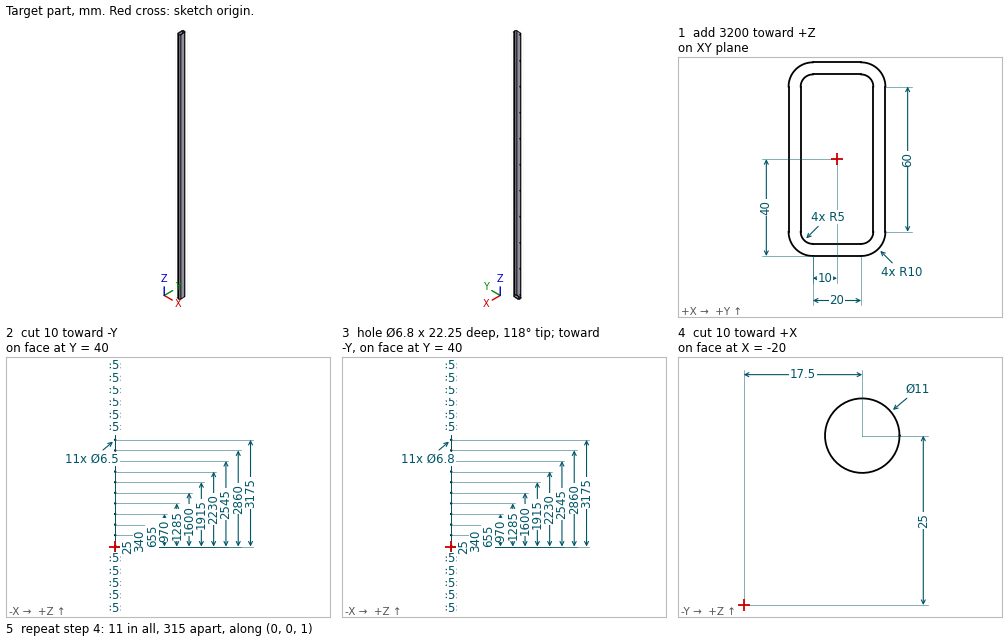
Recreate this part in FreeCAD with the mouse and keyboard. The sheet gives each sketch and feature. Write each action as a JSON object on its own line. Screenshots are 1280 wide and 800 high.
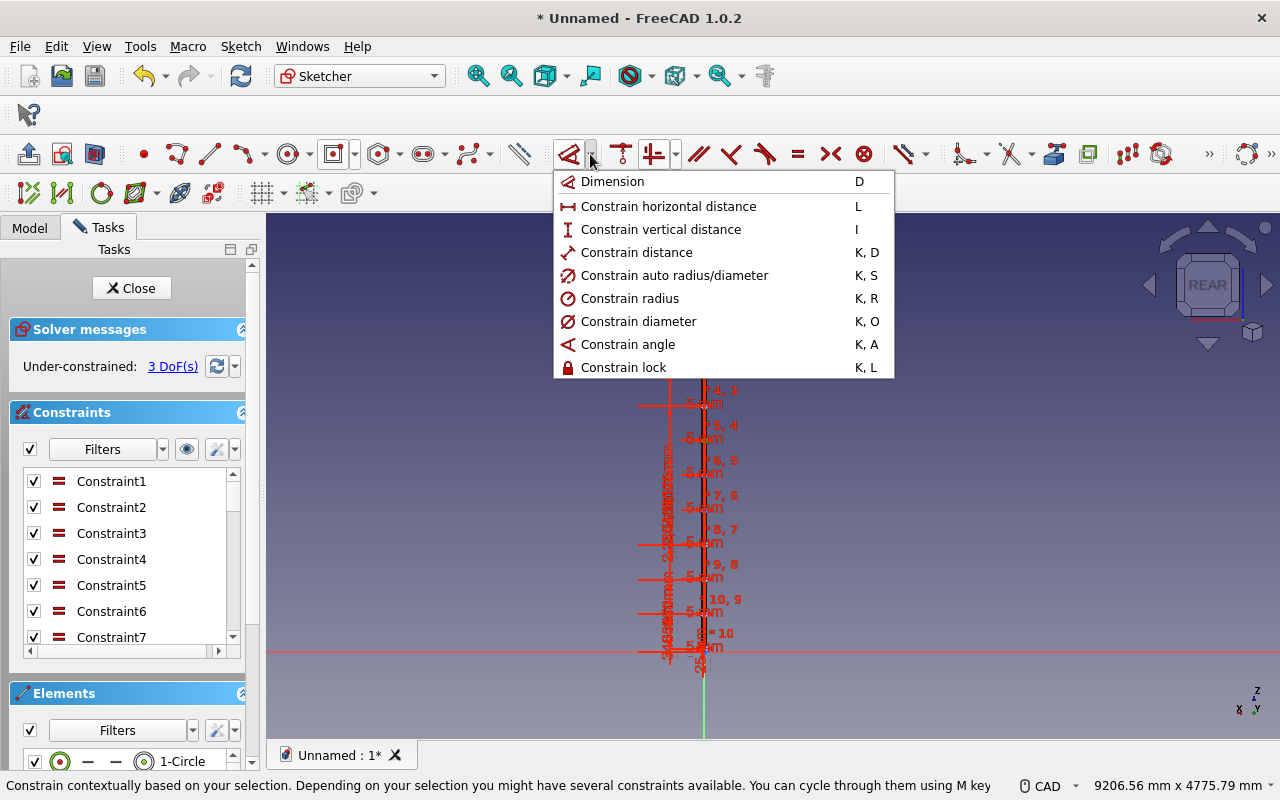
{"action": "left_click", "coordinate": [724, 230]}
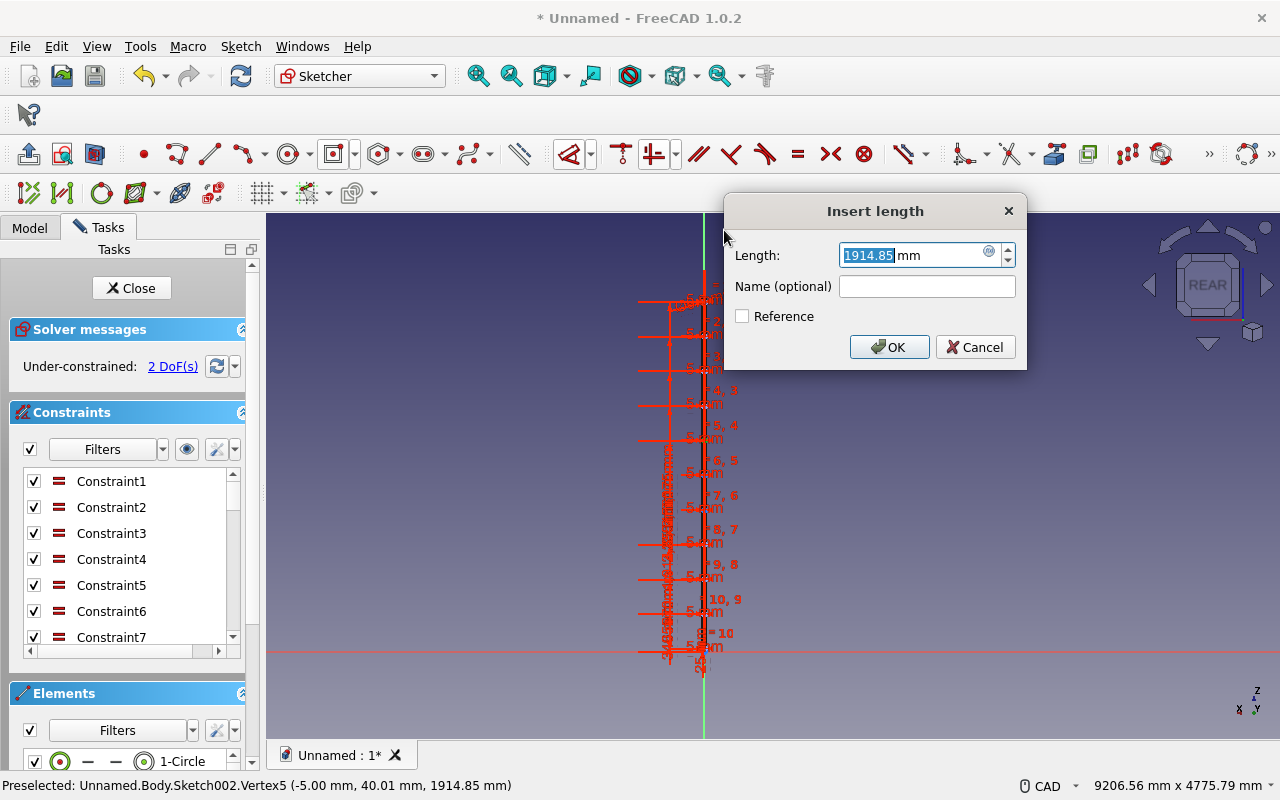
{"action": "type", "text": "1915"}
{"action": "key", "text": "Return"}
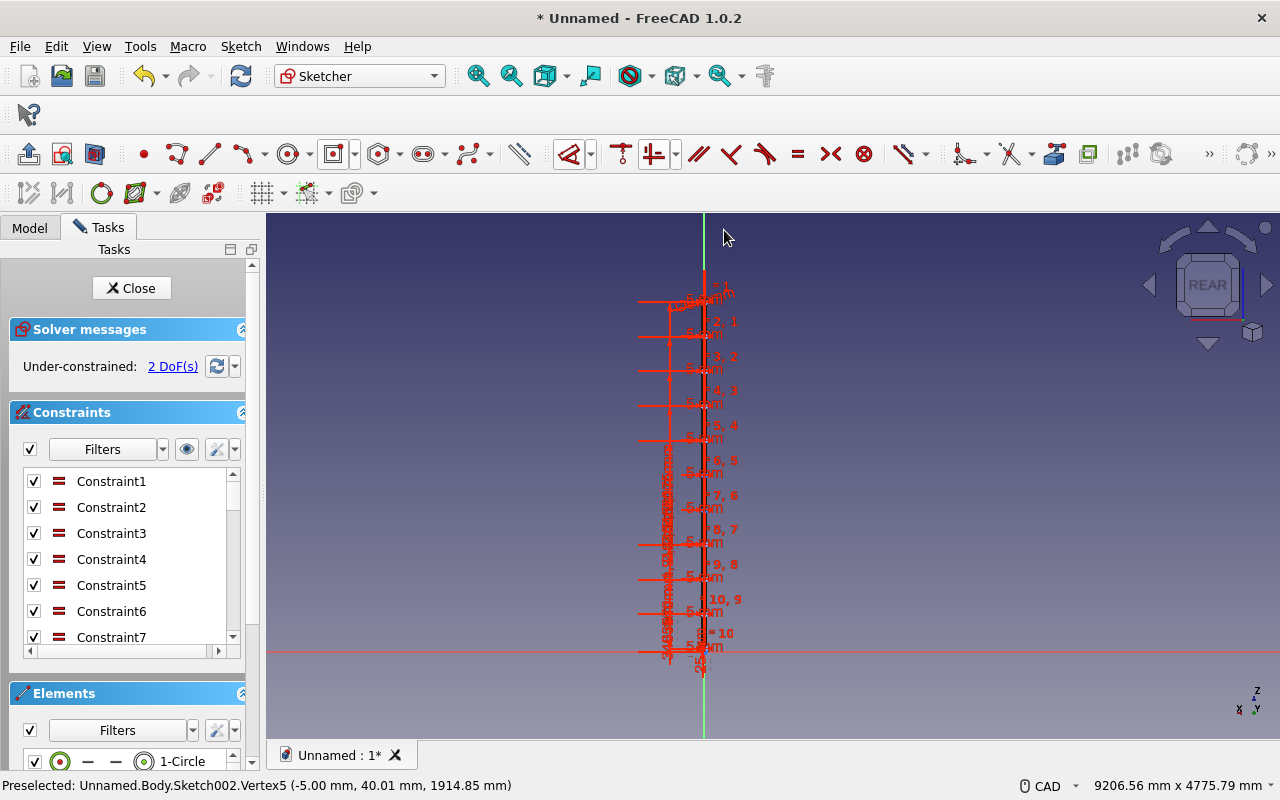
{"action": "left_click", "coordinate": [705, 476]}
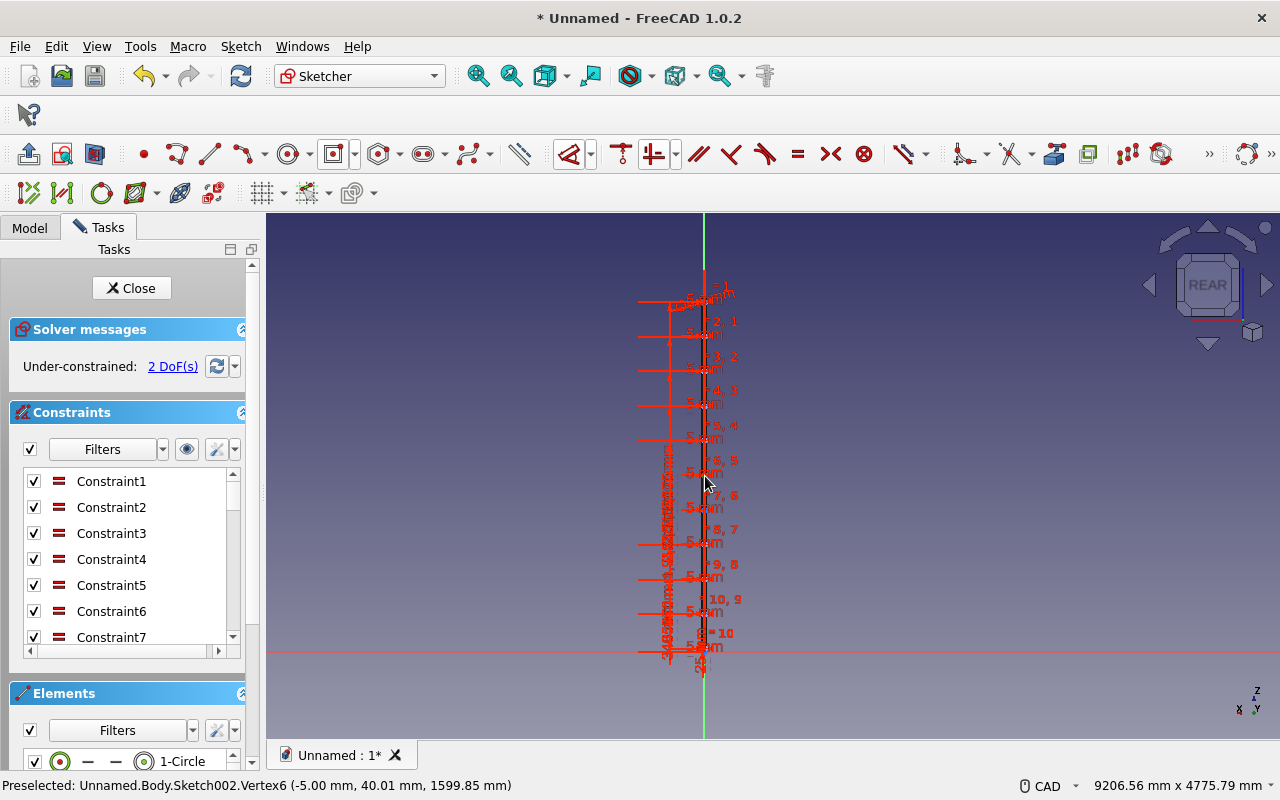
{"action": "key", "text": "i"}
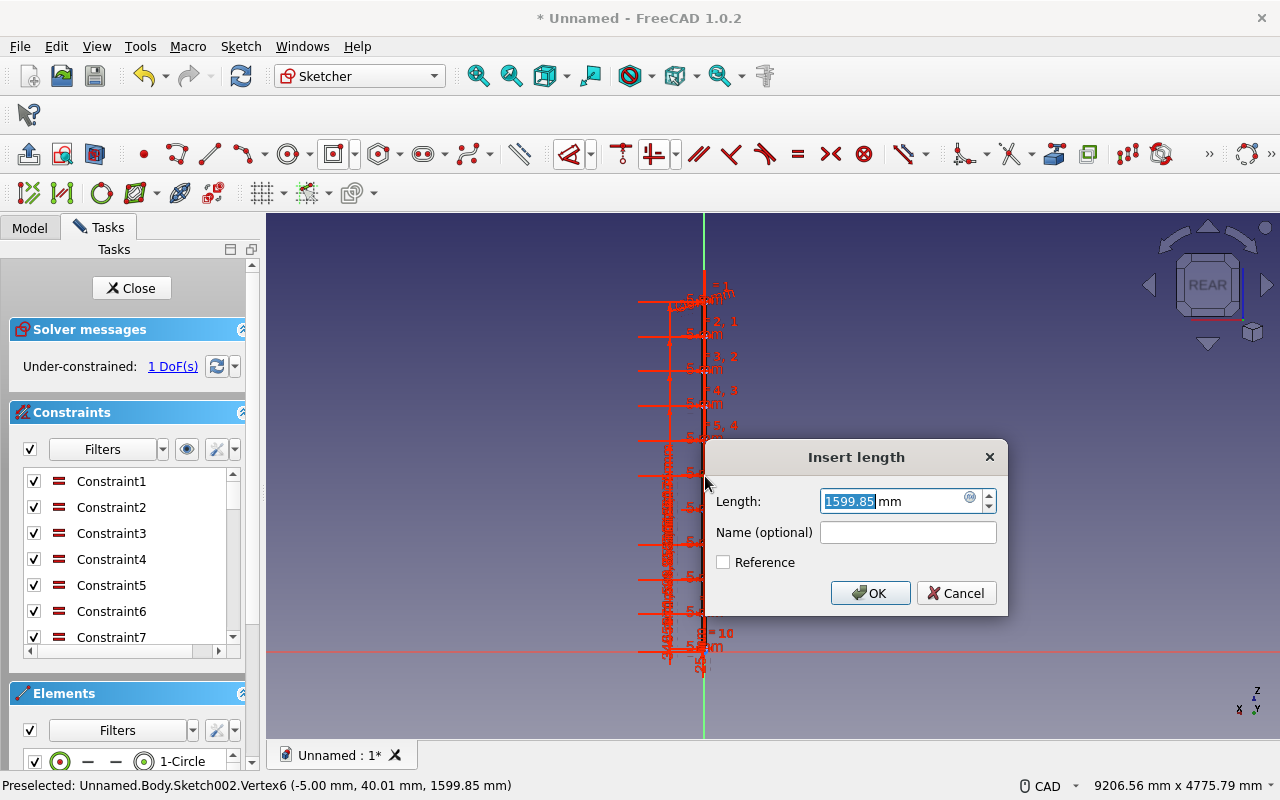
{"action": "type", "text": "1600"}
{"action": "key", "text": "Return"}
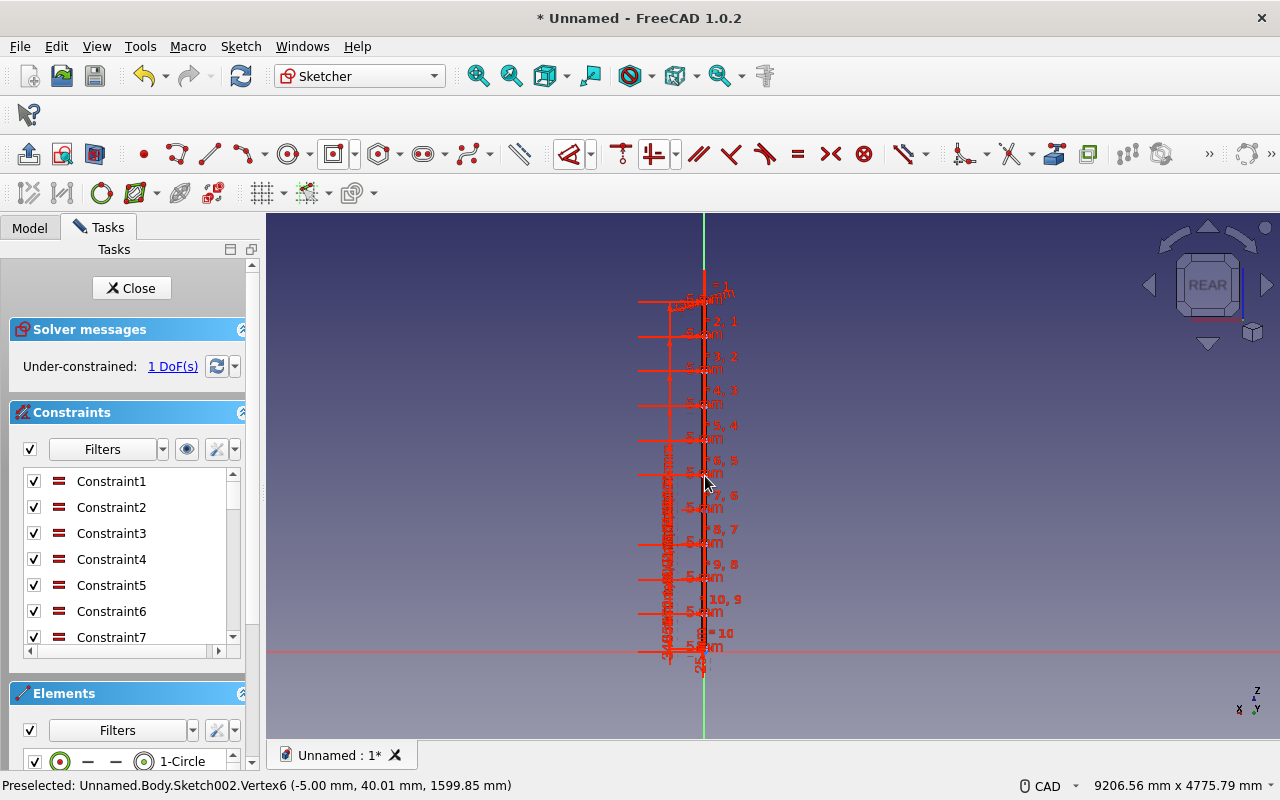
{"action": "left_click", "coordinate": [705, 510]}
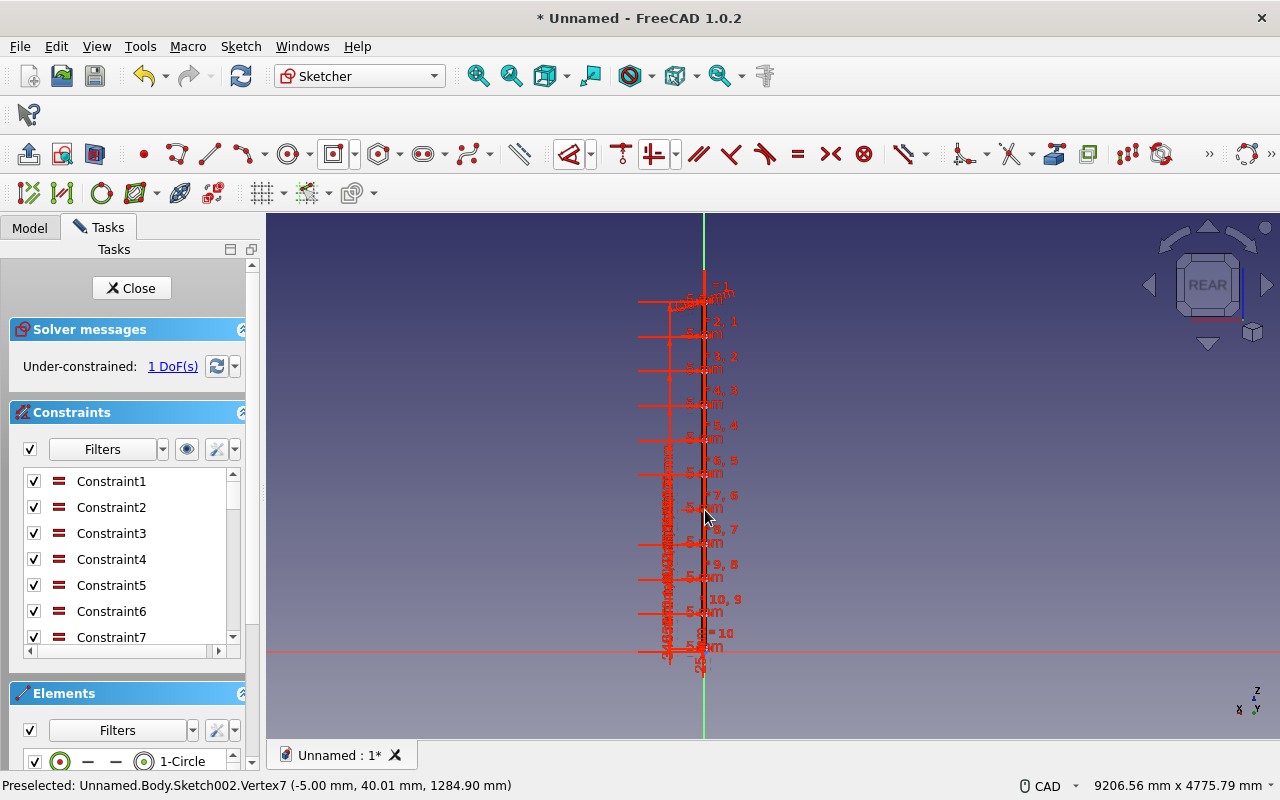
{"action": "left_click", "coordinate": [590, 154]}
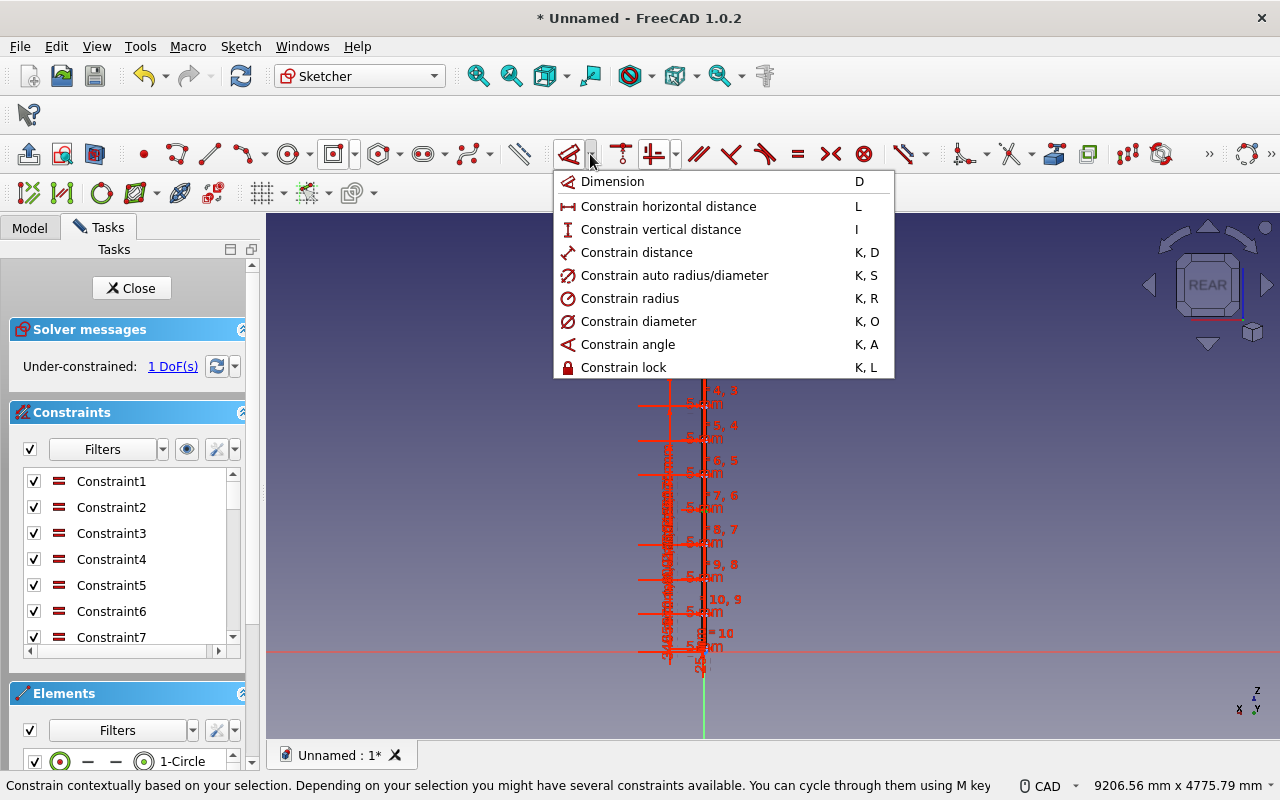
{"action": "left_click", "coordinate": [724, 230]}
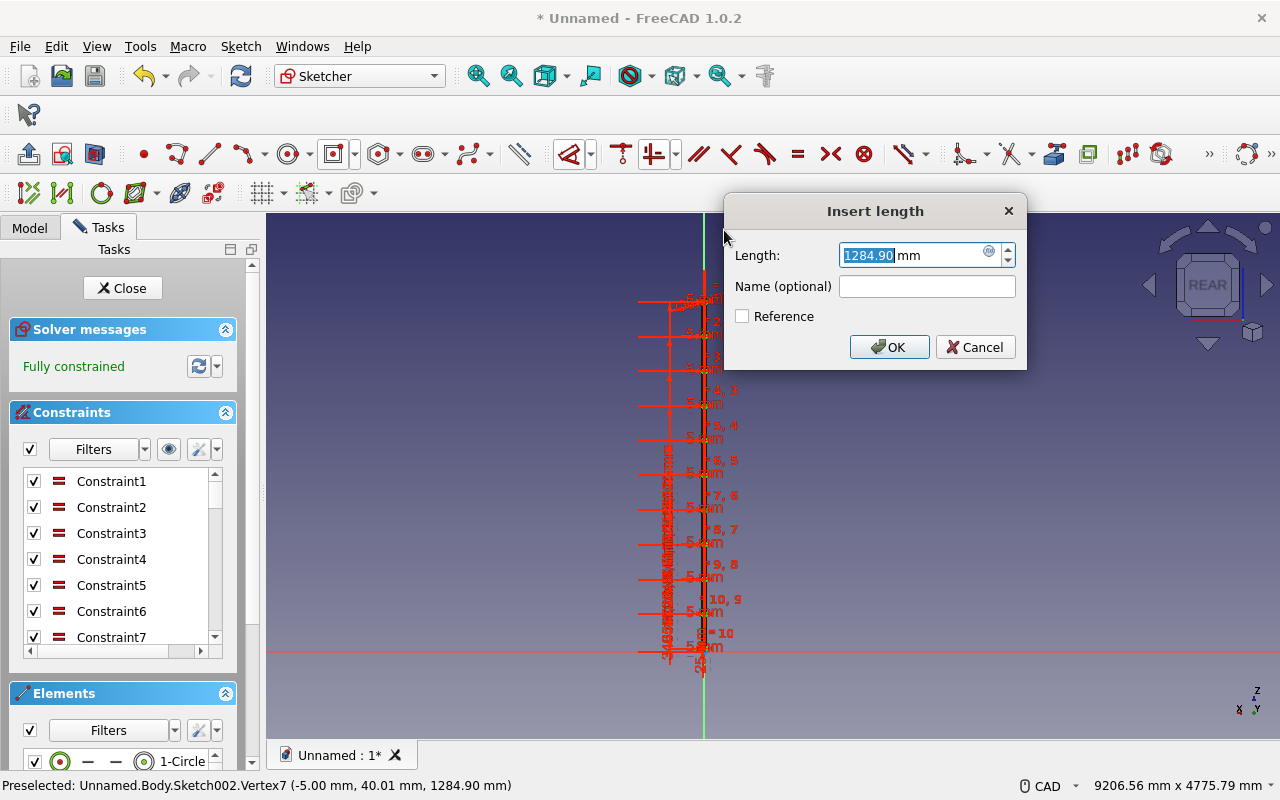
{"action": "type", "text": "1285"}
{"action": "key", "text": "Return"}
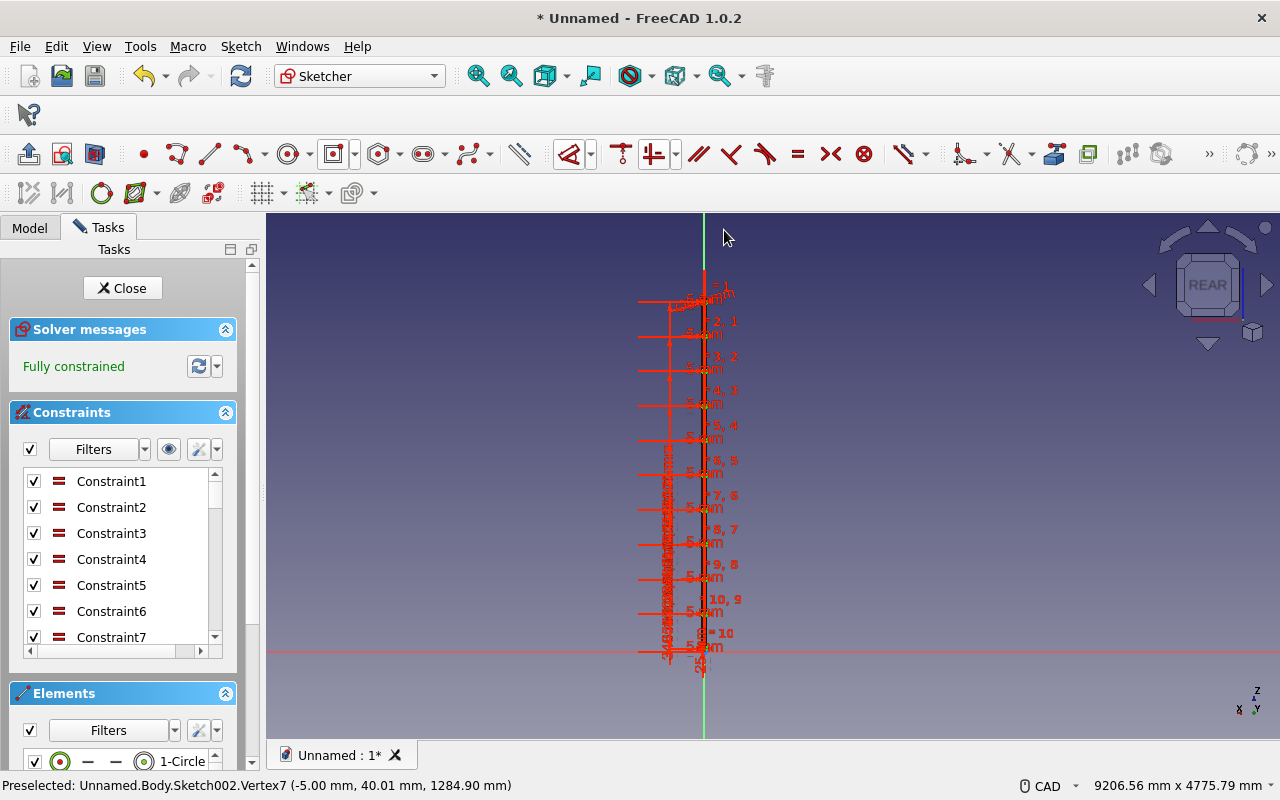
{"action": "left_click", "coordinate": [123, 288]}